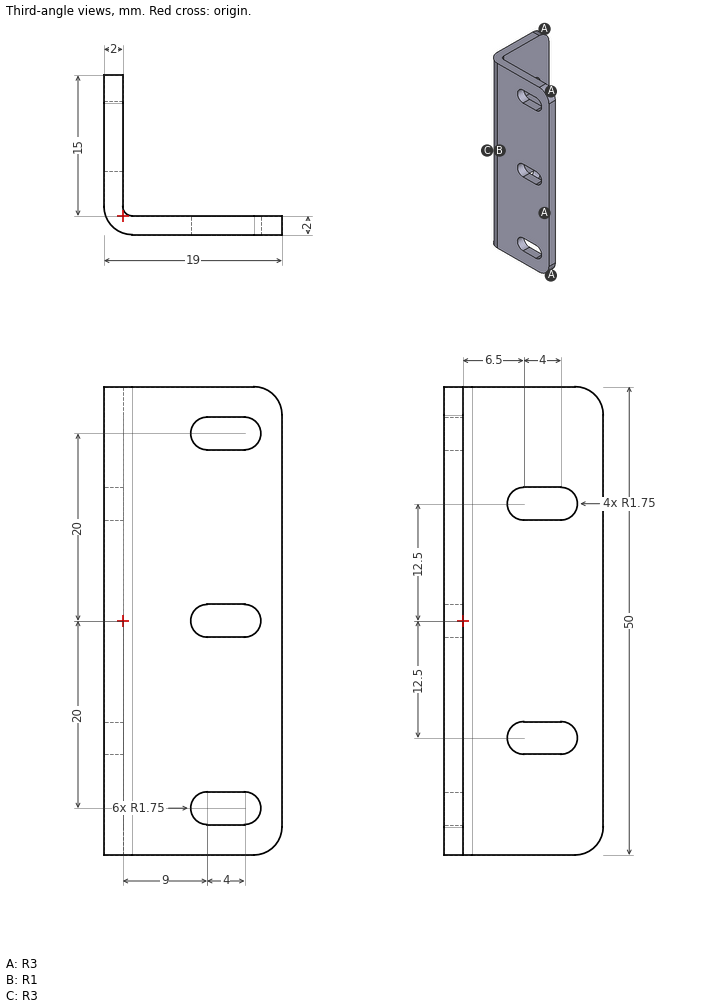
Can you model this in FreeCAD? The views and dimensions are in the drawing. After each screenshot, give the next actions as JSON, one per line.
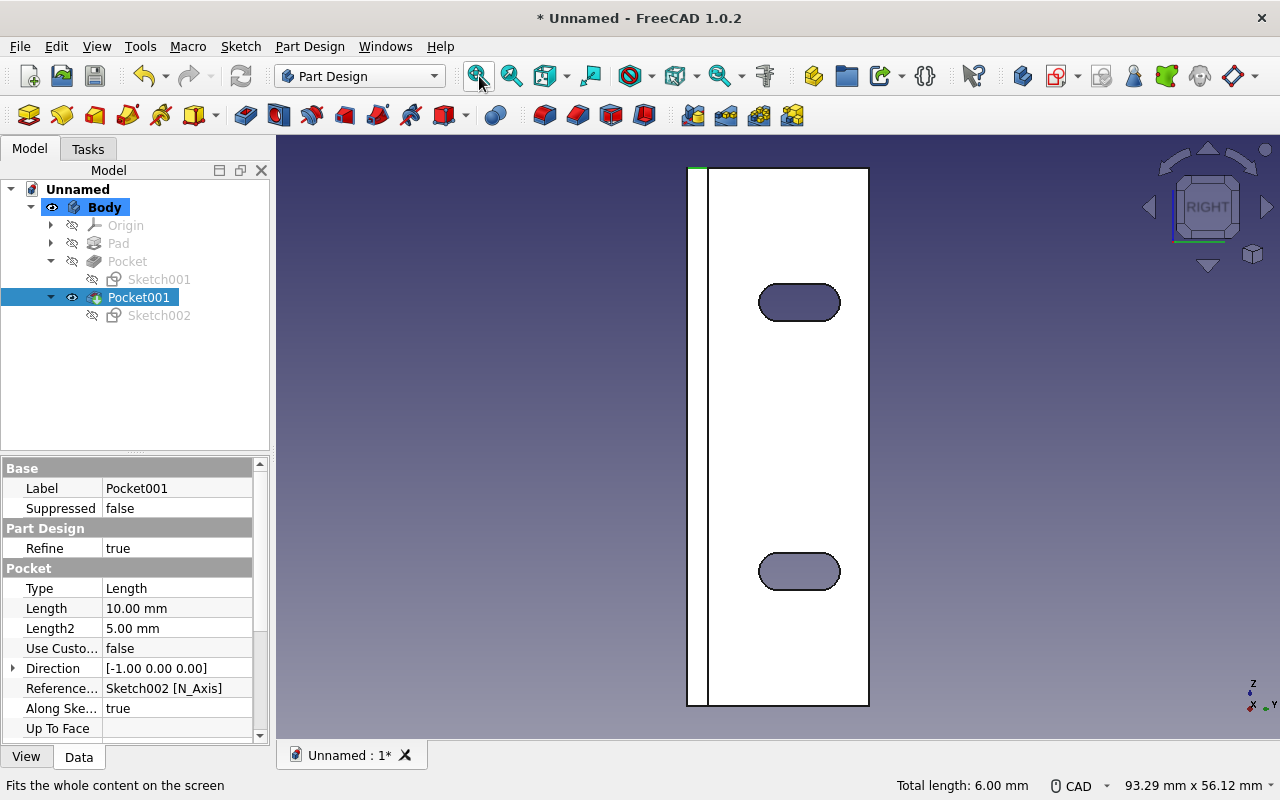
{"action": "left_click", "coordinate": [697, 705], "text": "ctrl"}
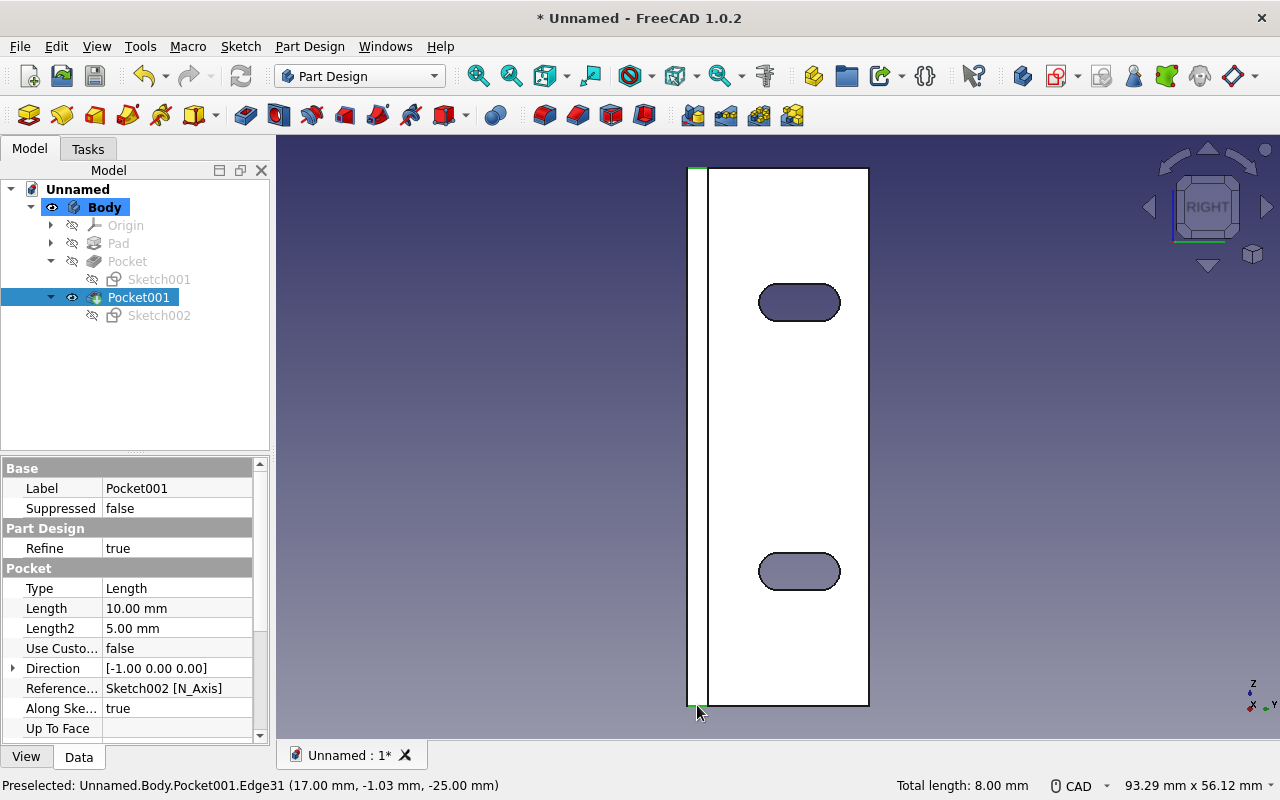
{"action": "left_click", "coordinate": [545, 116]}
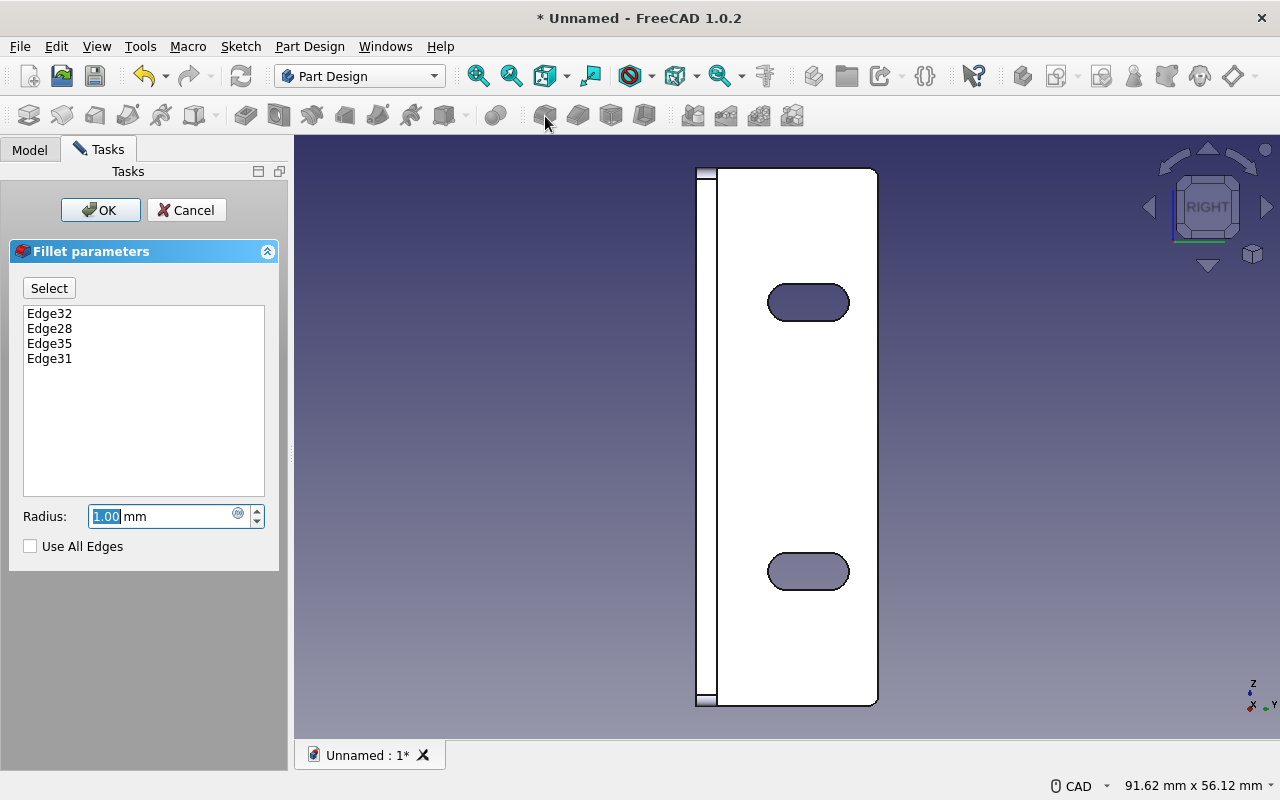
{"action": "type", "text": "3"}
{"action": "key", "text": "Tab"}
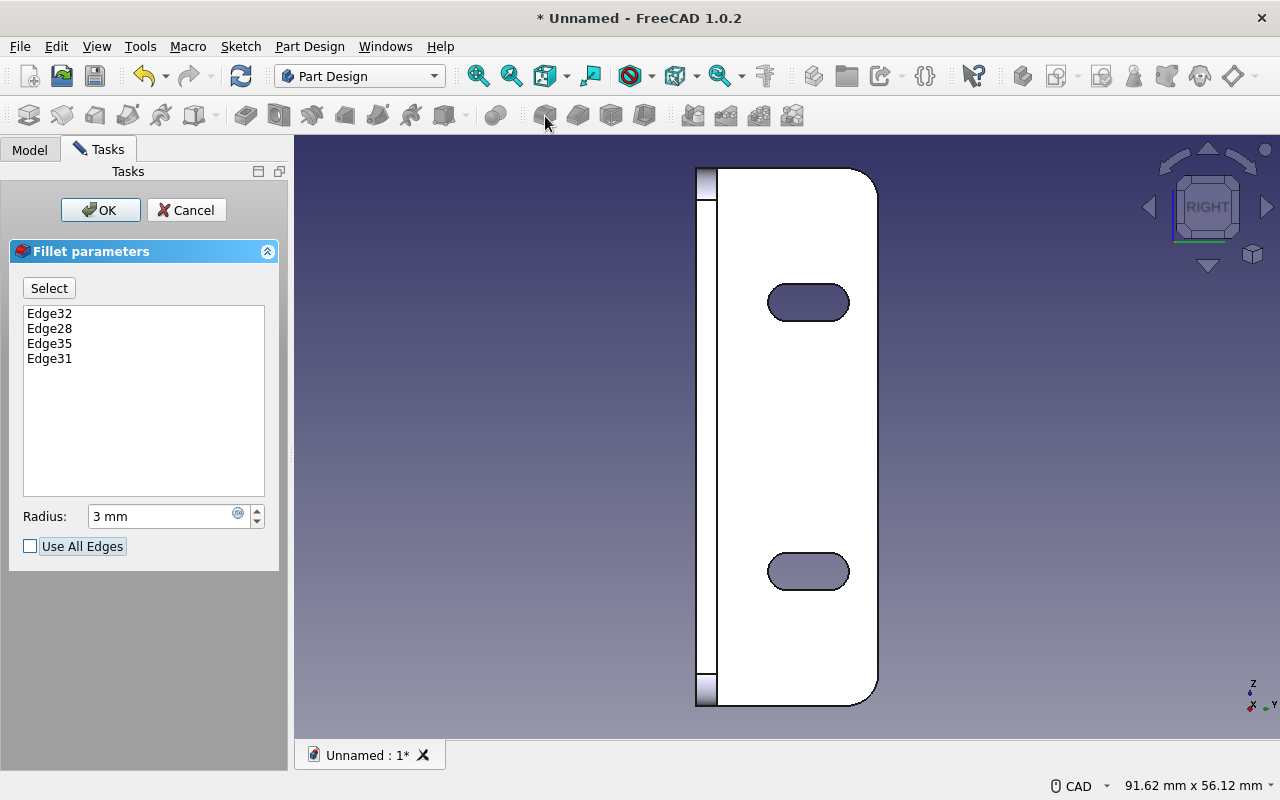
{"action": "left_click", "coordinate": [101, 210]}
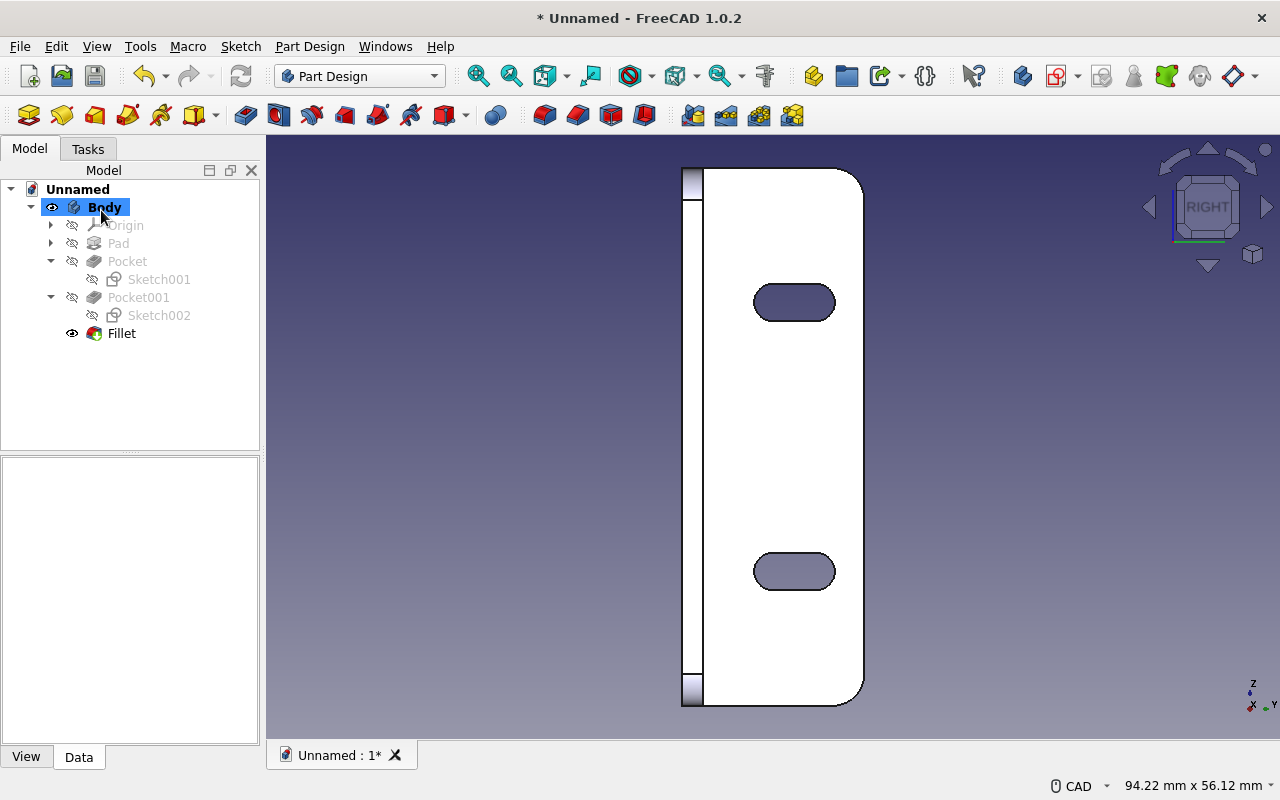
{"action": "key", "text": "0"}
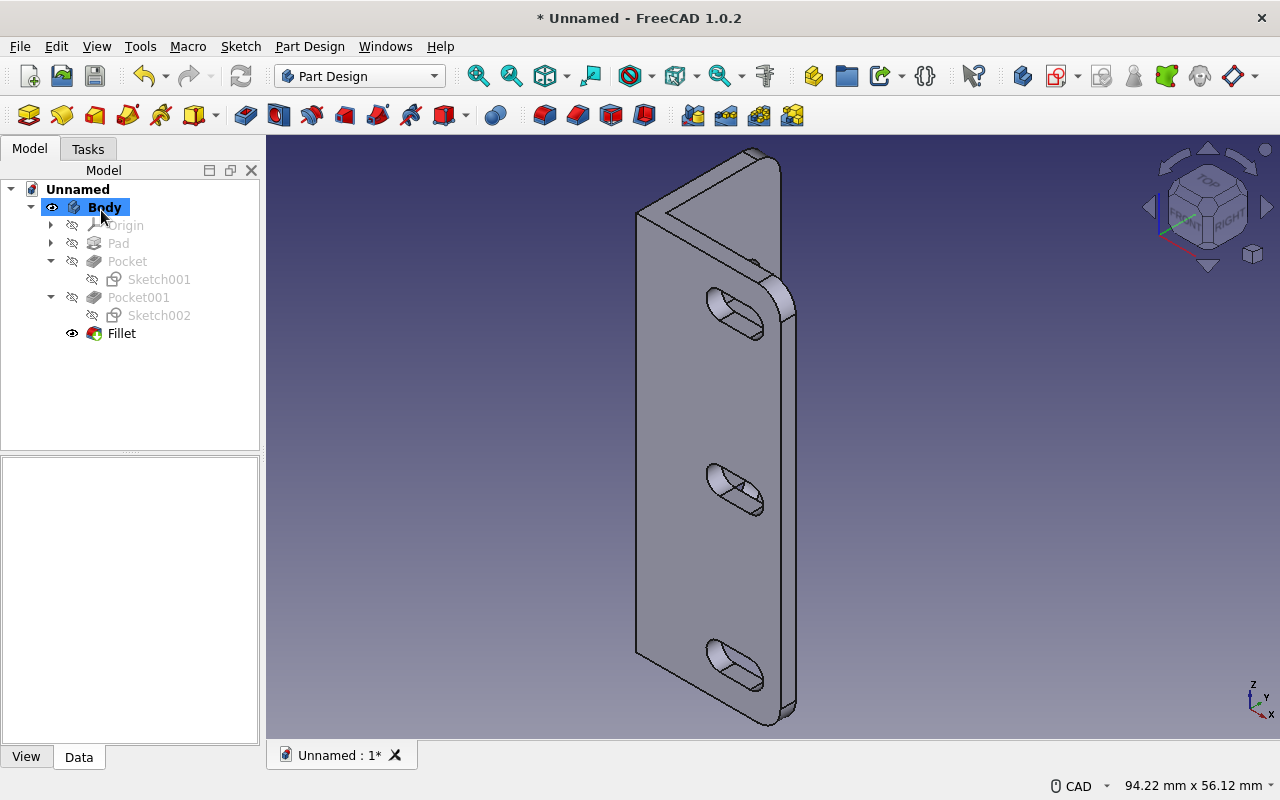
{"action": "key", "text": "2"}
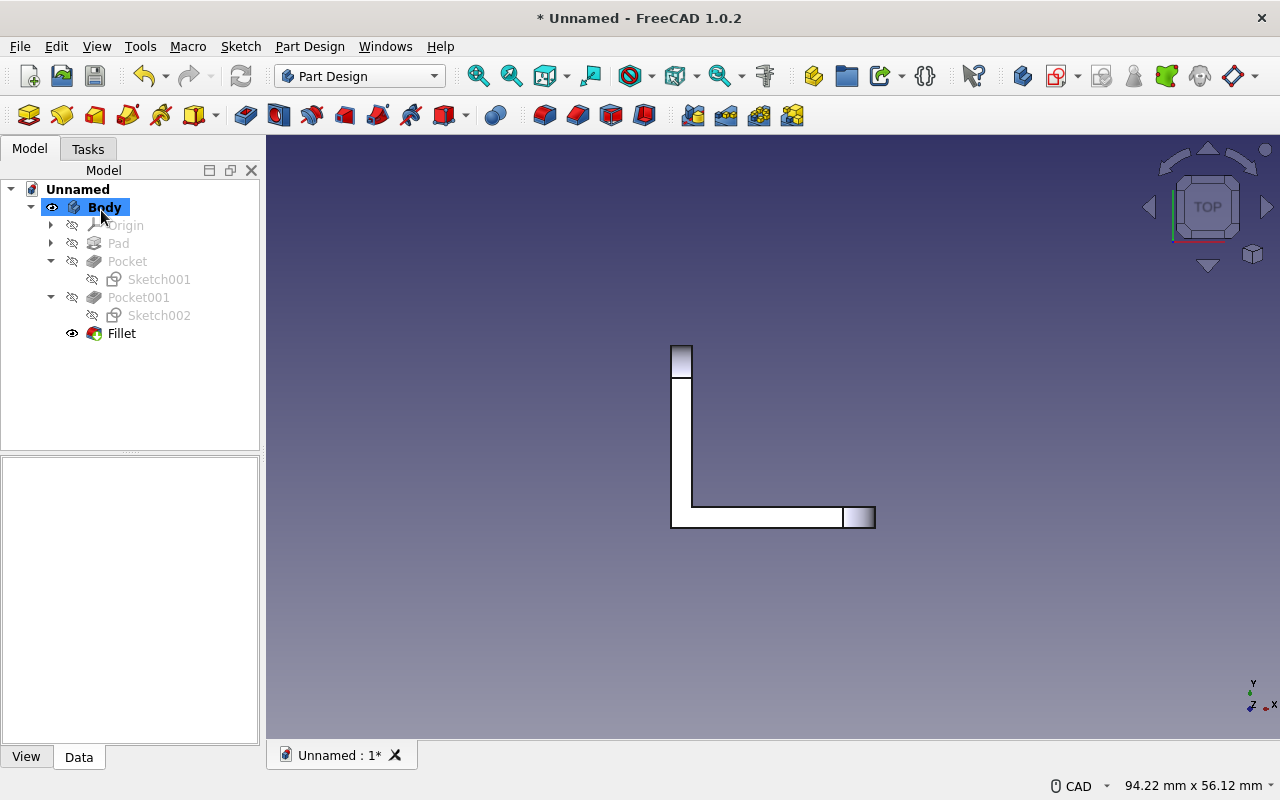
{"action": "left_click", "coordinate": [479, 76]}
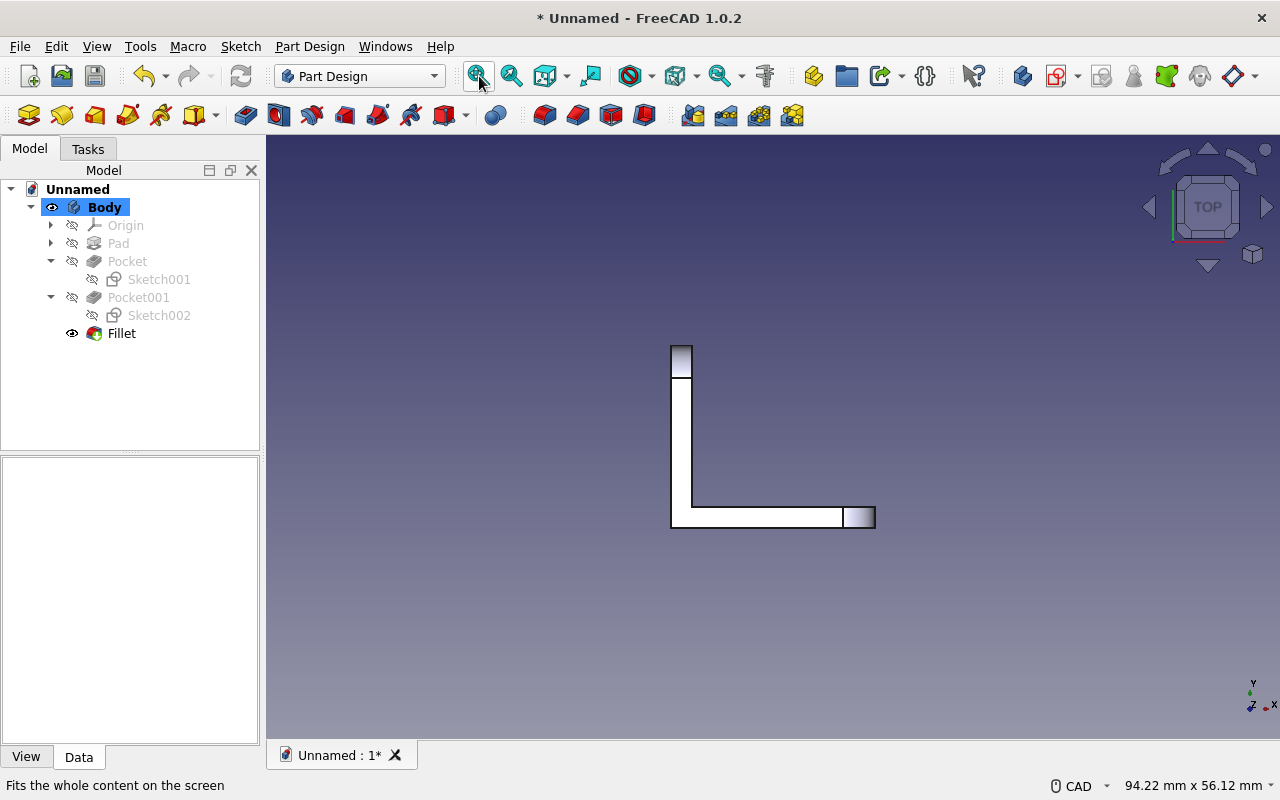
{"action": "key", "text": "1"}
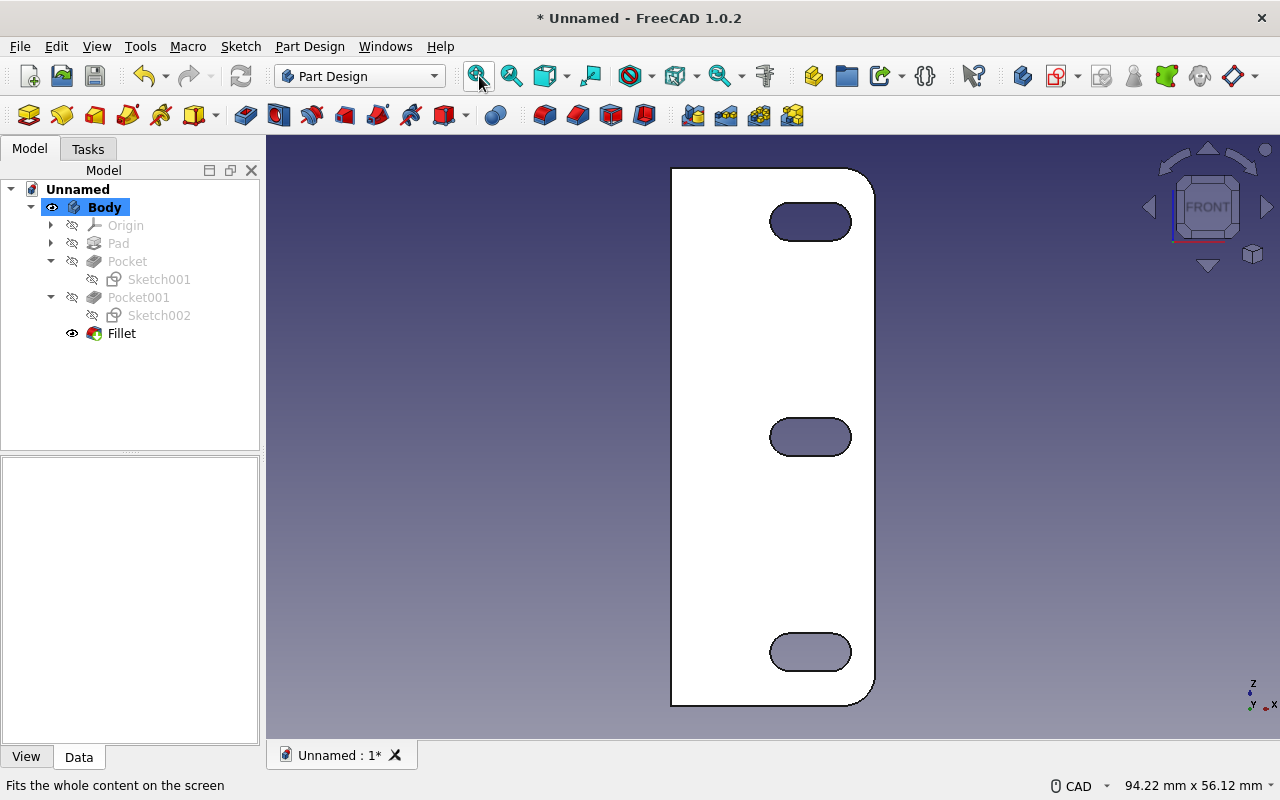
{"action": "key", "text": "3"}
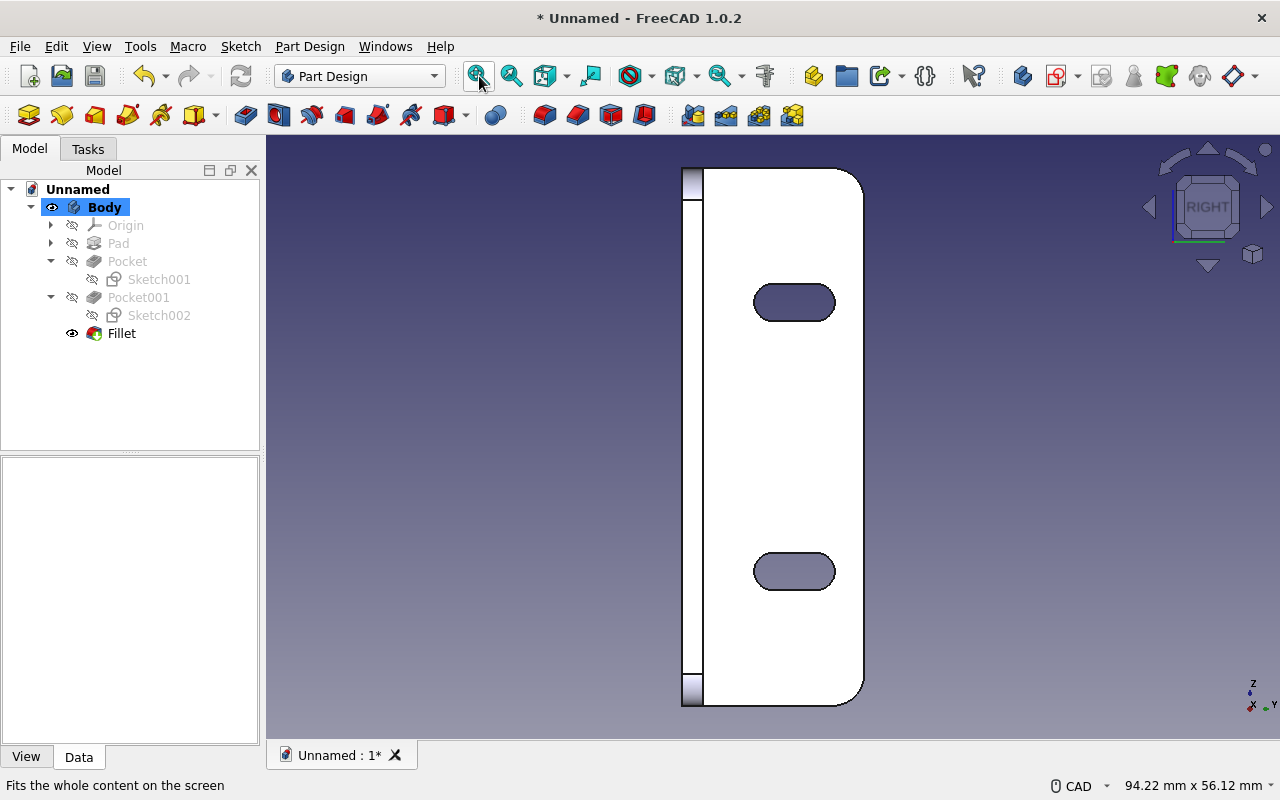
{"action": "key", "text": "5"}